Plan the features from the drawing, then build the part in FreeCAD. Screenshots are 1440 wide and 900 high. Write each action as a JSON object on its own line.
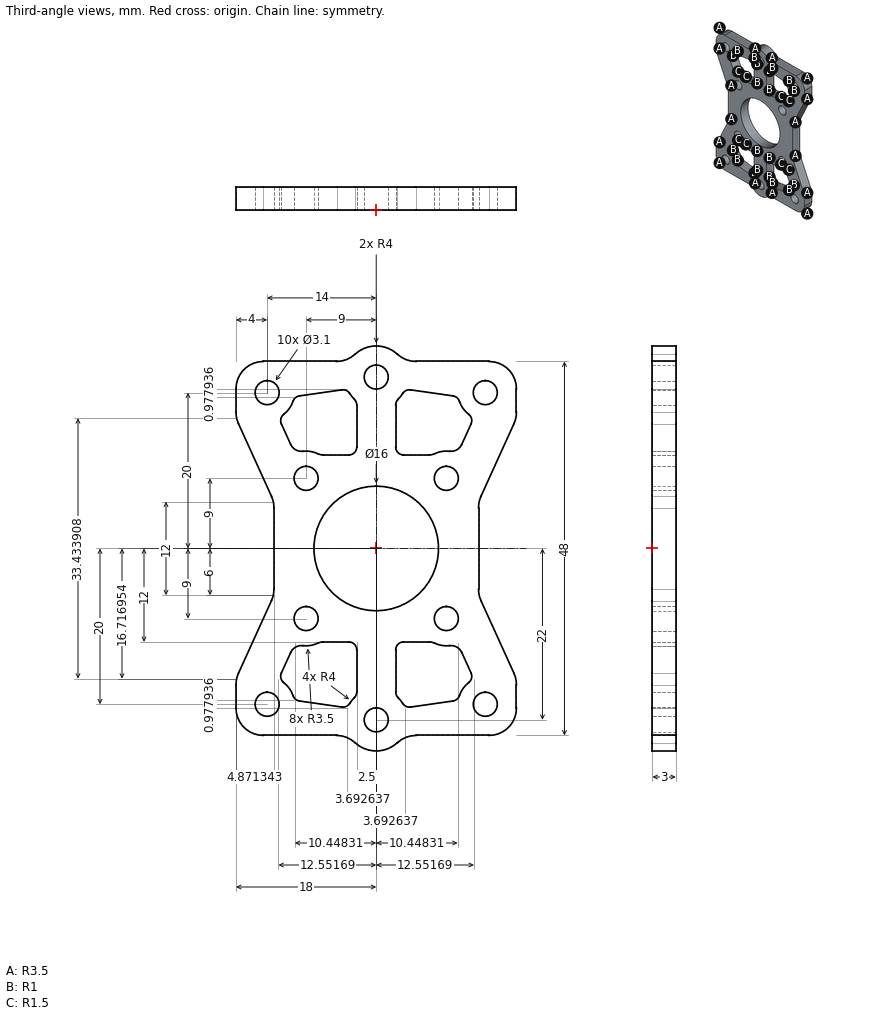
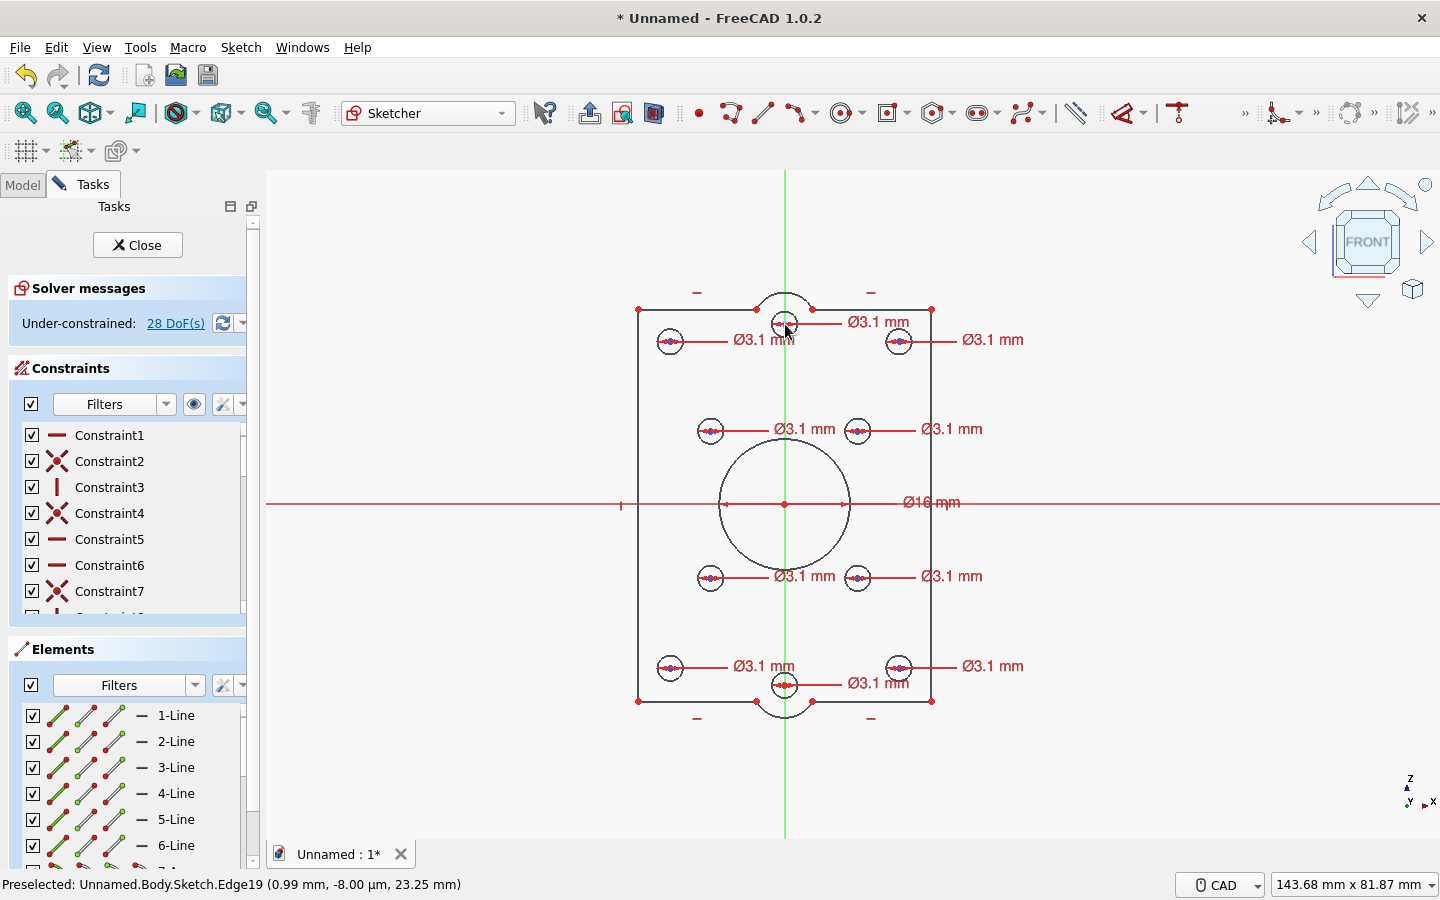
{"action": "left_click", "coordinate": [771, 715]}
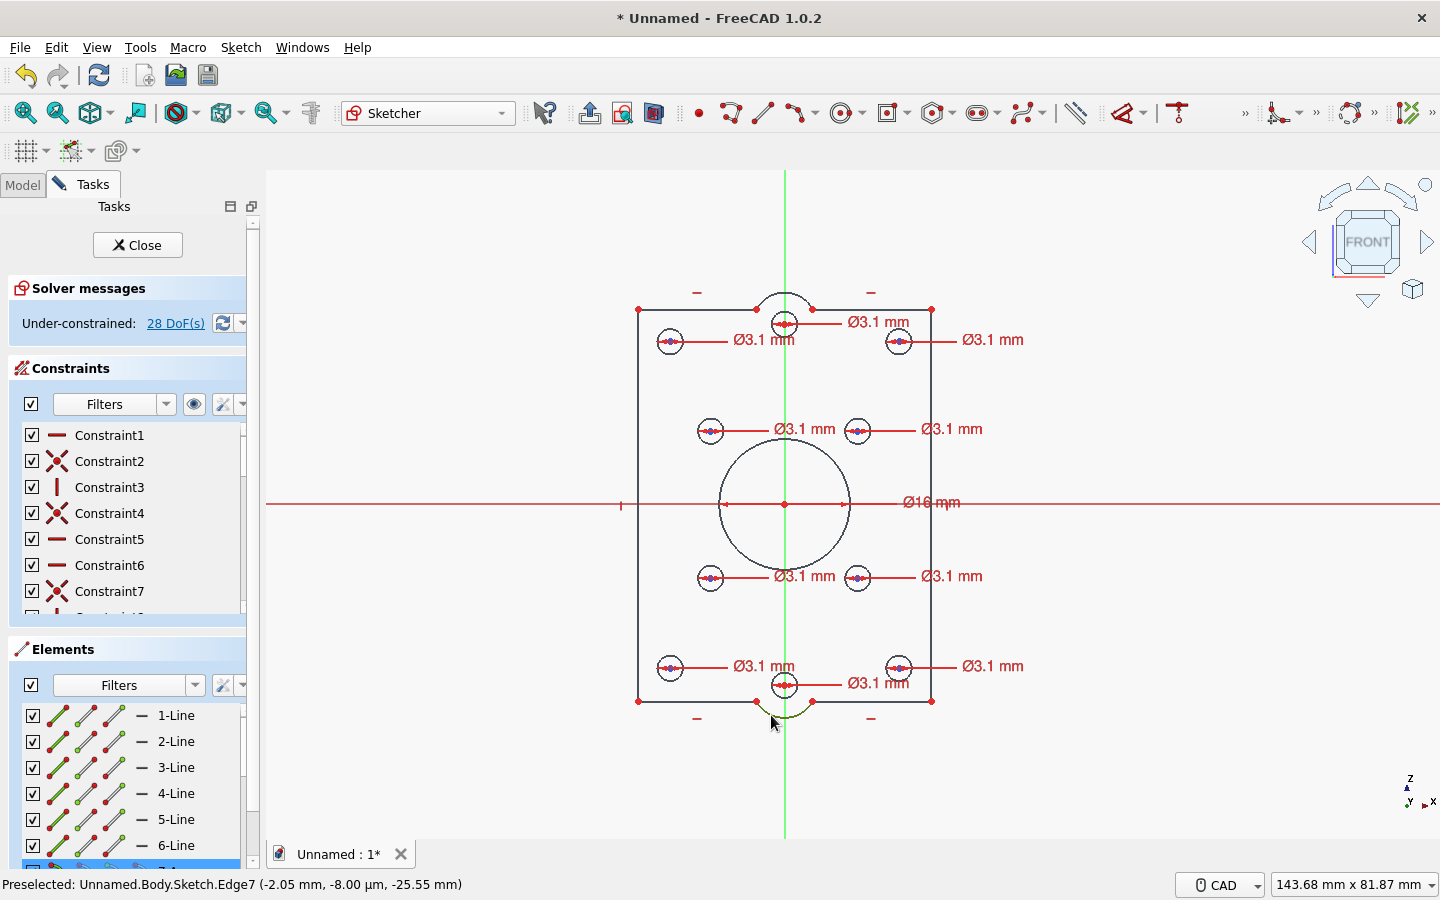
{"action": "left_click", "coordinate": [798, 296]}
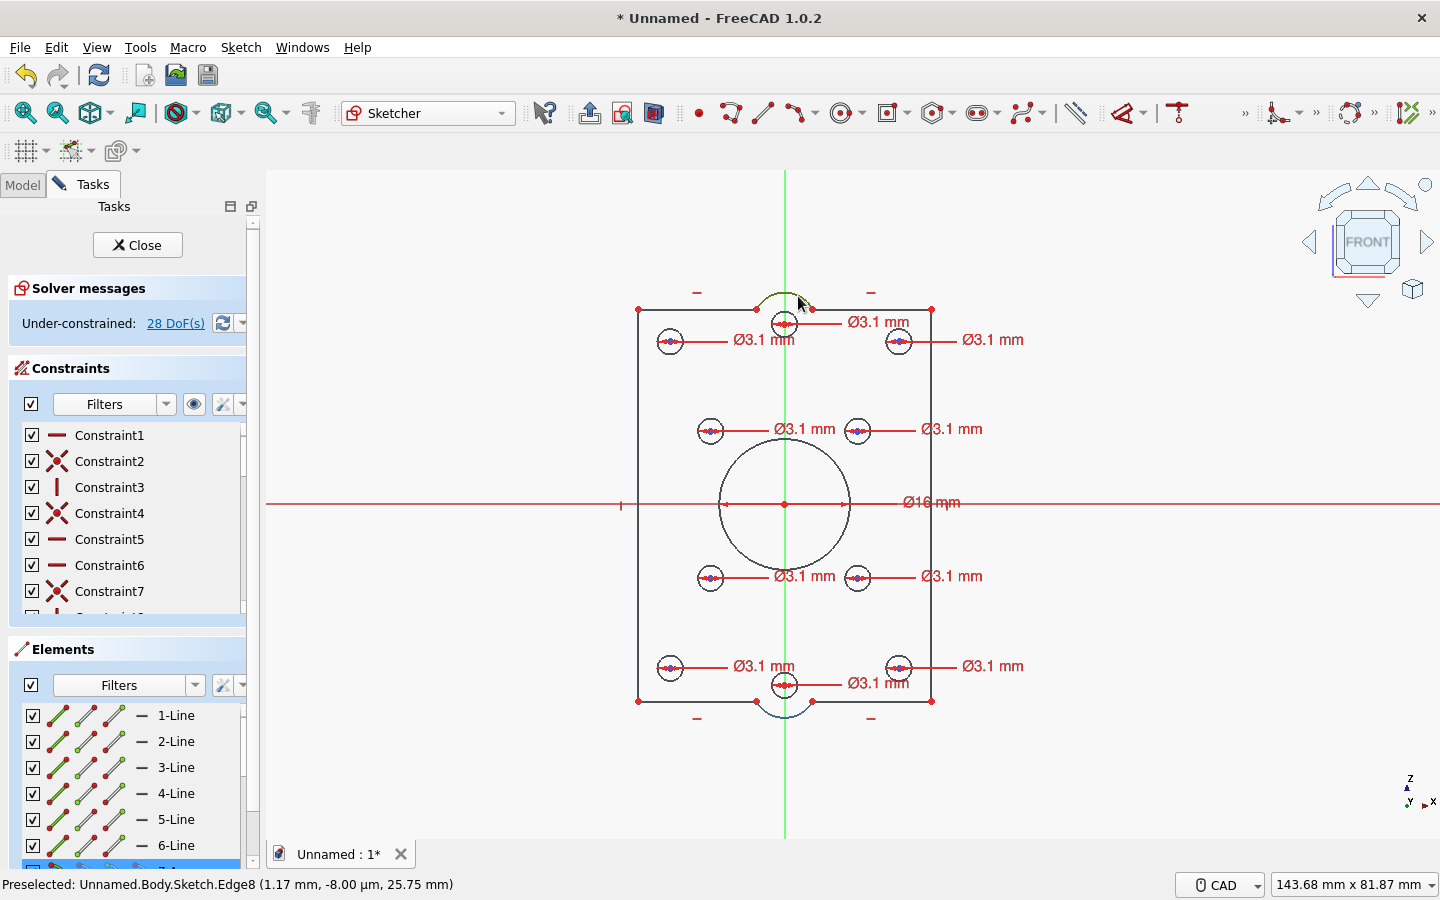
{"action": "key", "text": "e"}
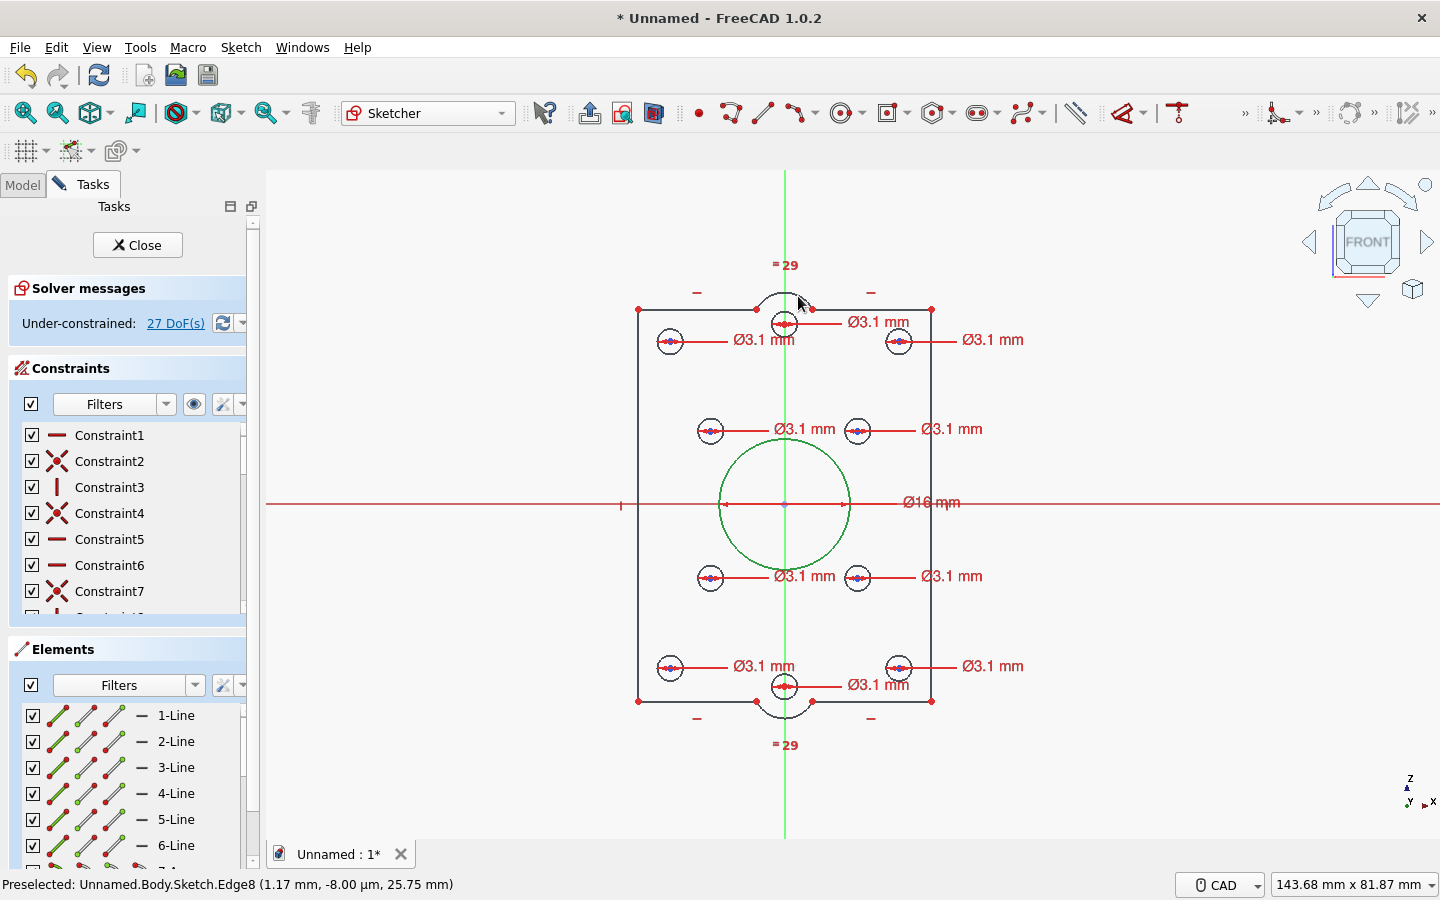
{"action": "left_click", "coordinate": [785, 687]}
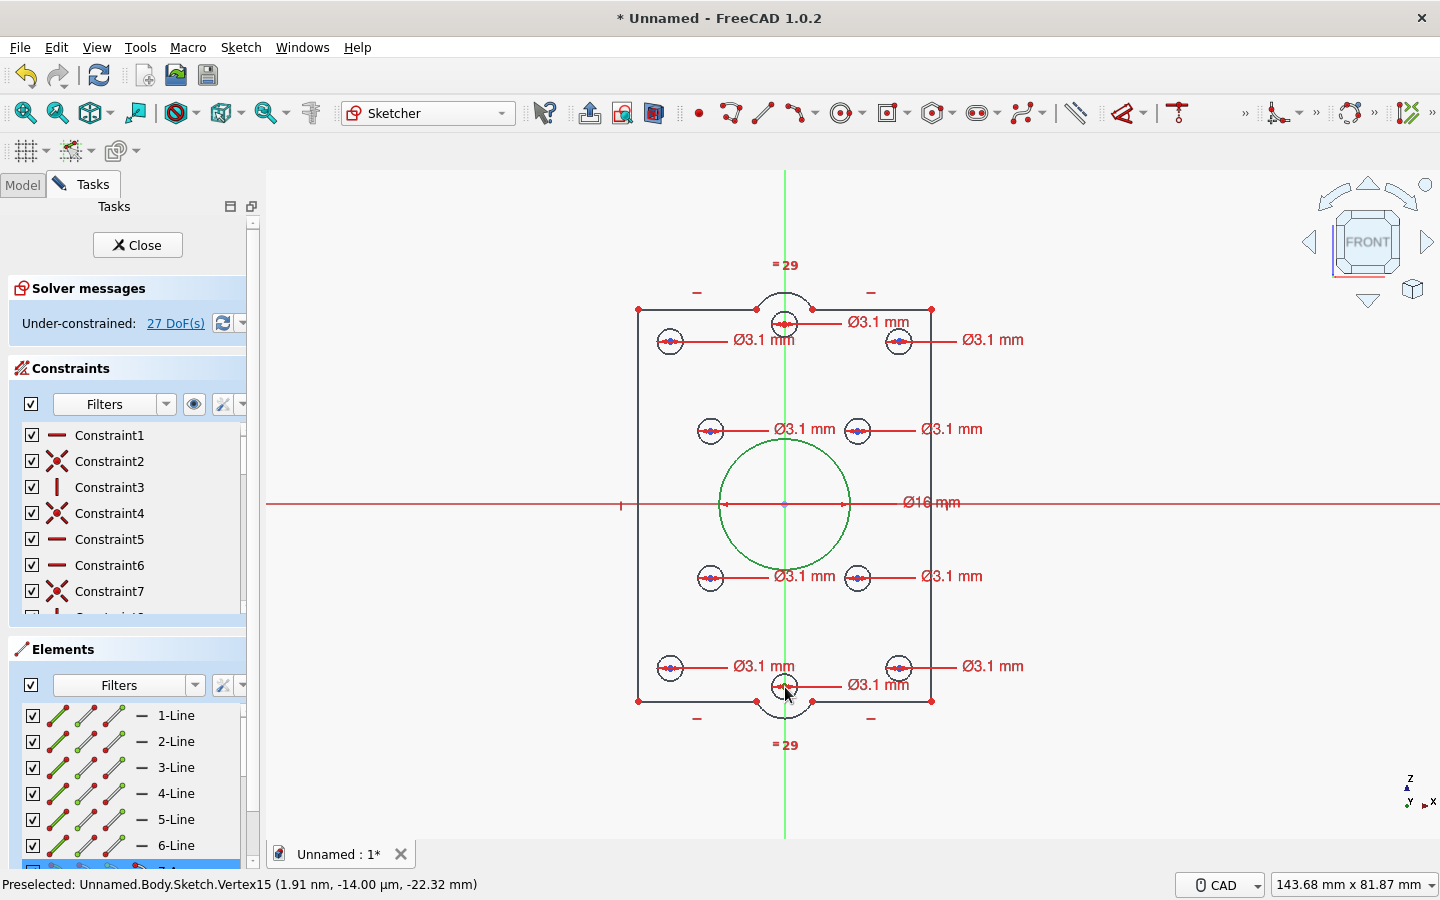
{"action": "left_click", "coordinate": [785, 767]}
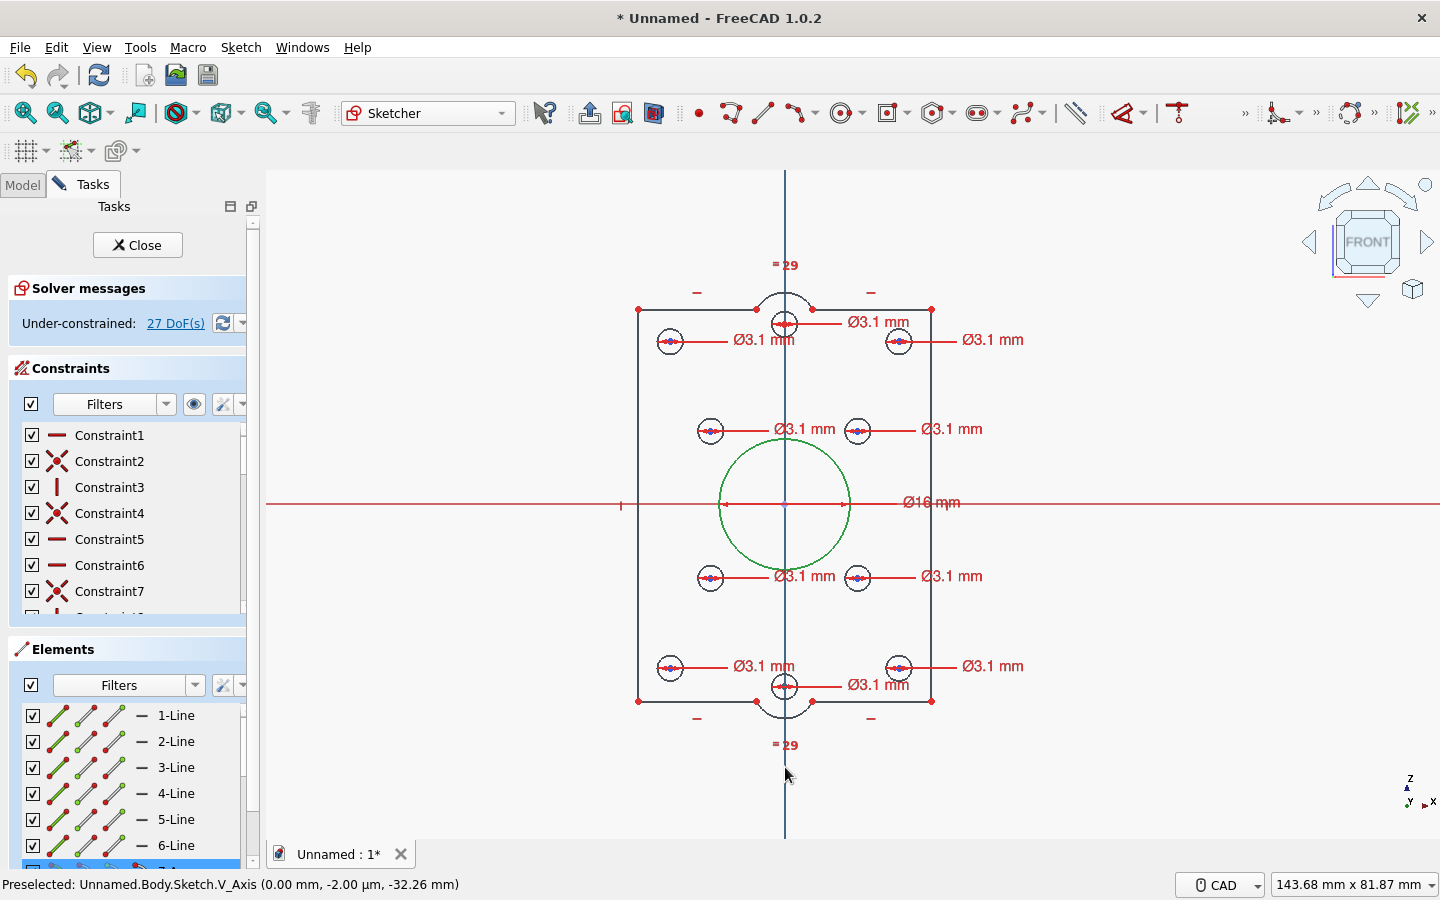
{"action": "left_click", "coordinate": [1178, 114]}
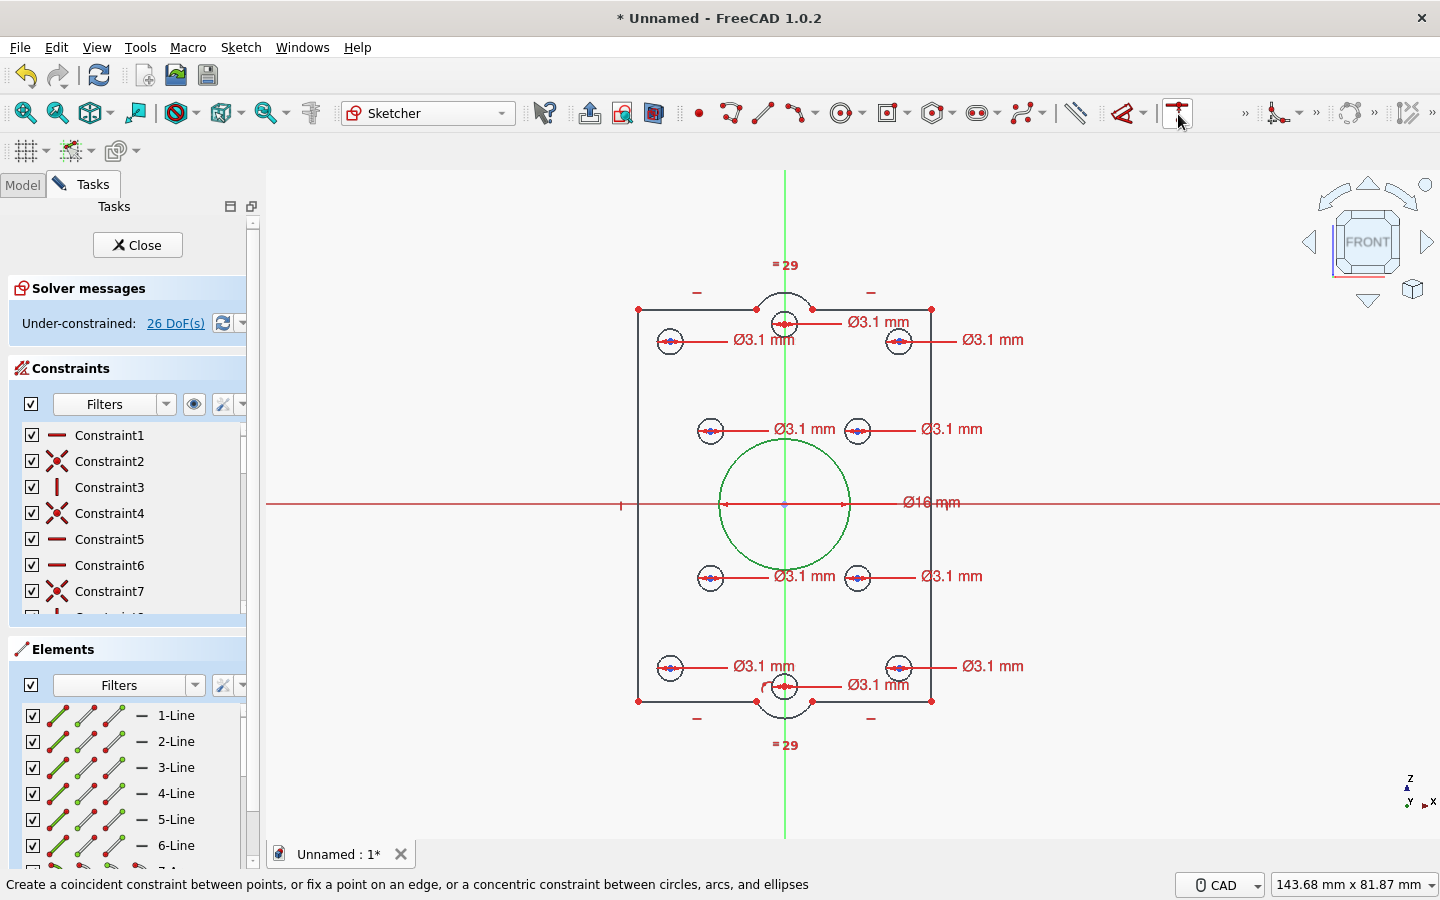
{"action": "left_click", "coordinate": [785, 324]}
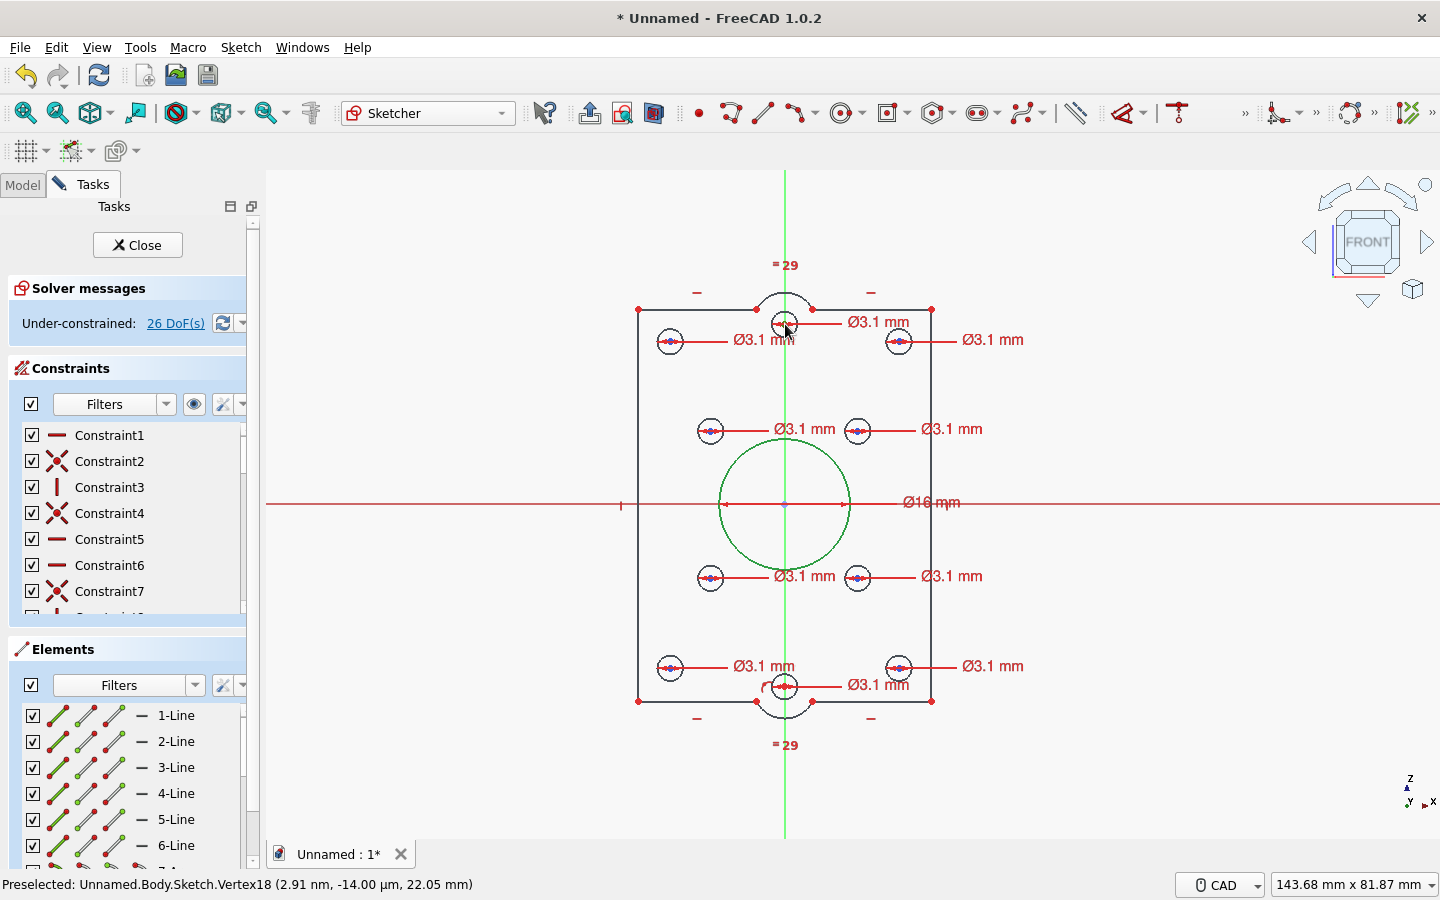
{"action": "left_click", "coordinate": [785, 767]}